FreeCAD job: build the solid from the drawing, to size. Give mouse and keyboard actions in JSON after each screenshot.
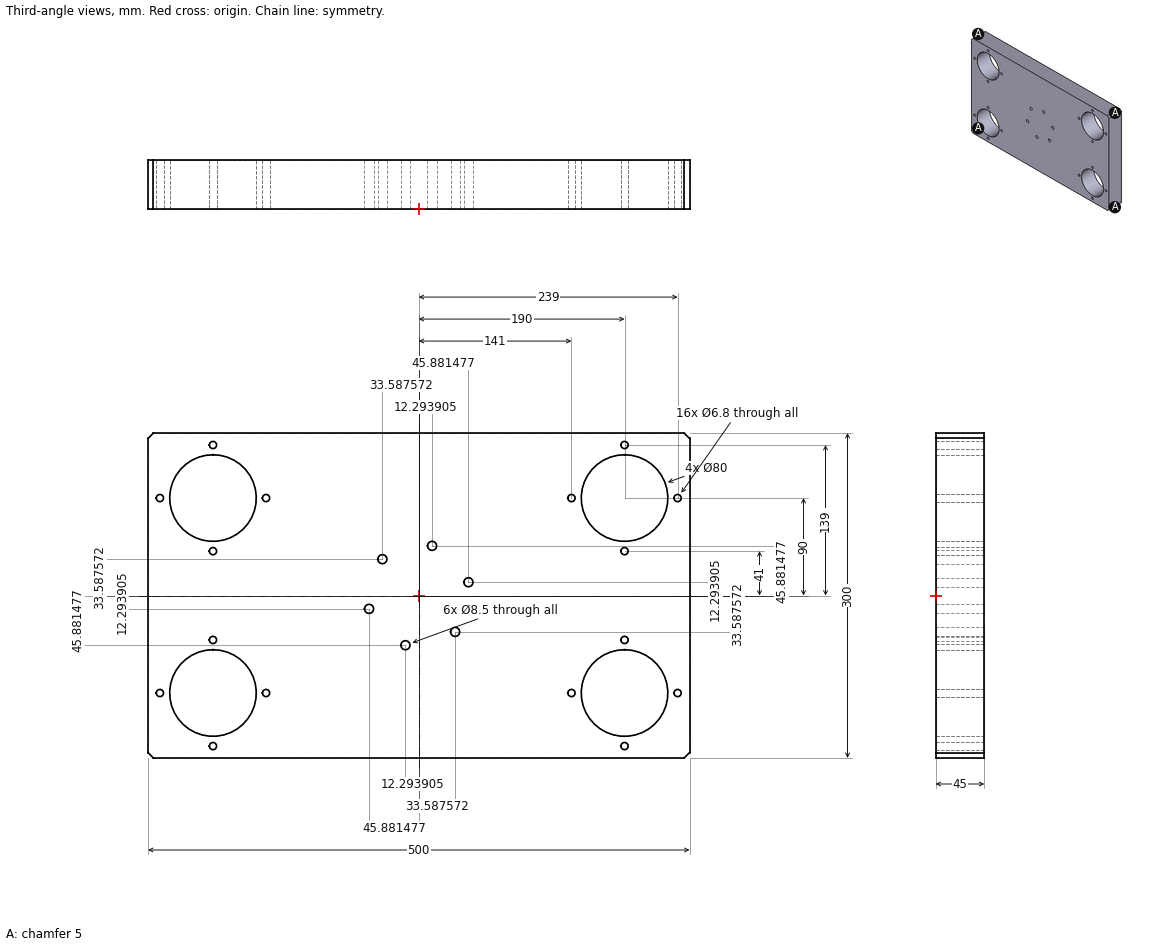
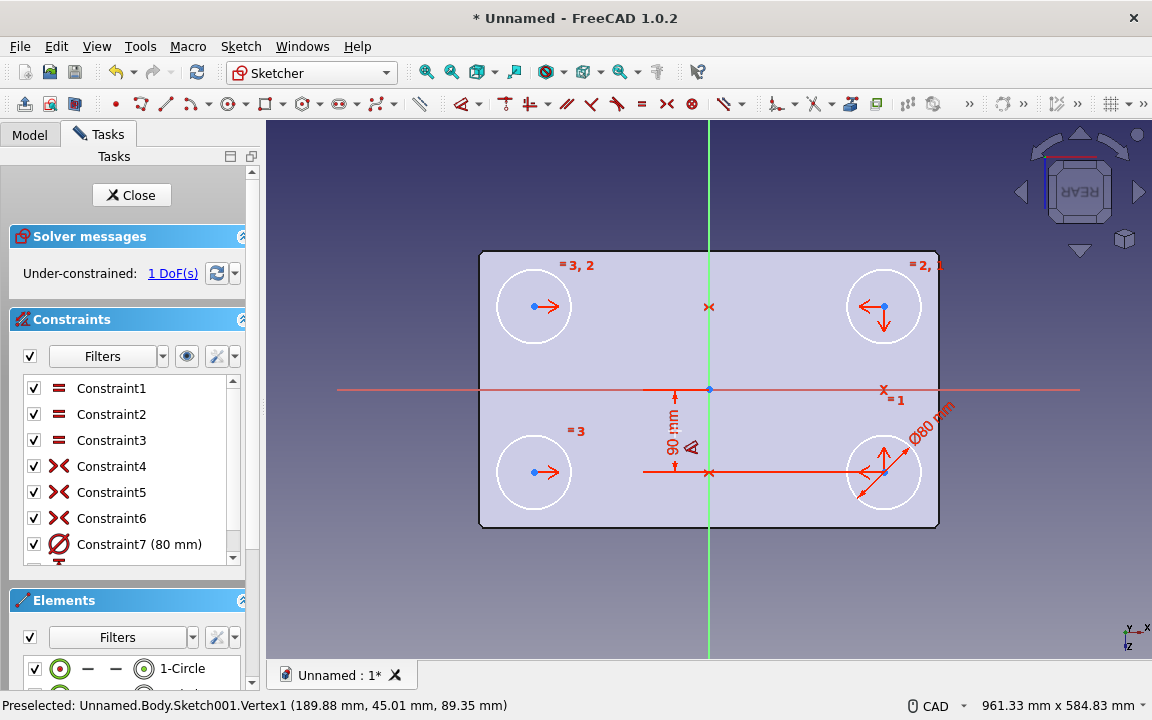
{"action": "left_click", "coordinate": [884, 472]}
{"action": "left_click", "coordinate": [796, 506]}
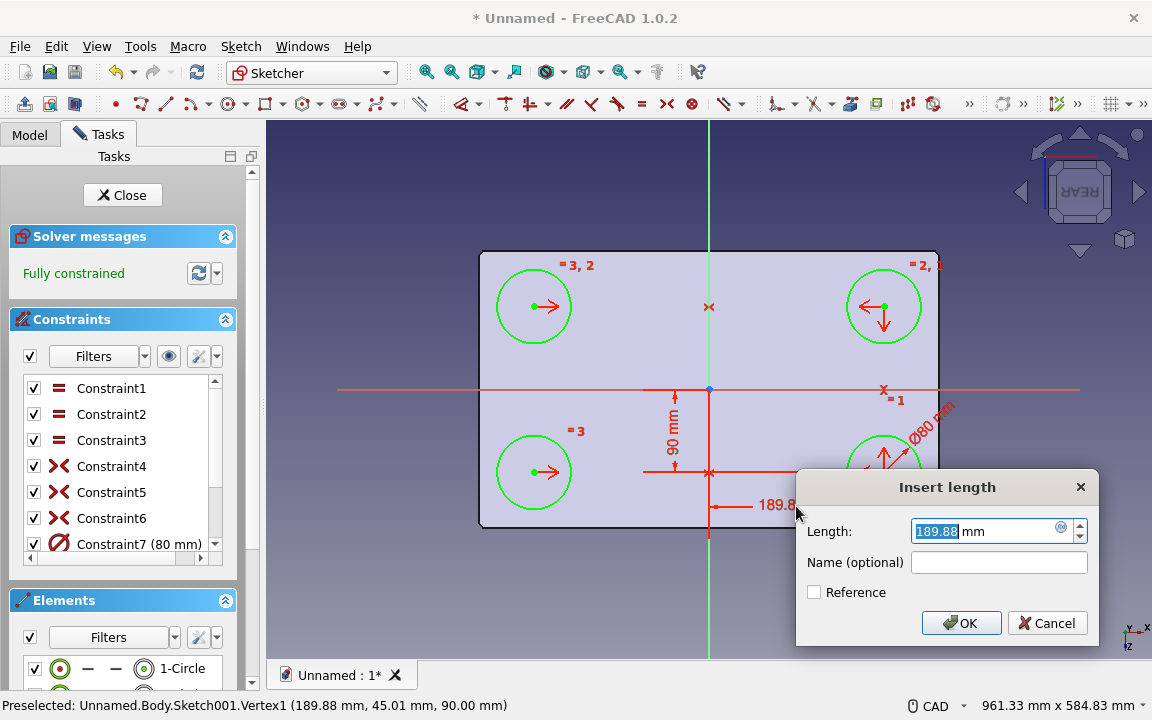
{"action": "type", "text": "190"}
{"action": "key", "text": "Return"}
{"action": "key", "text": "Escape"}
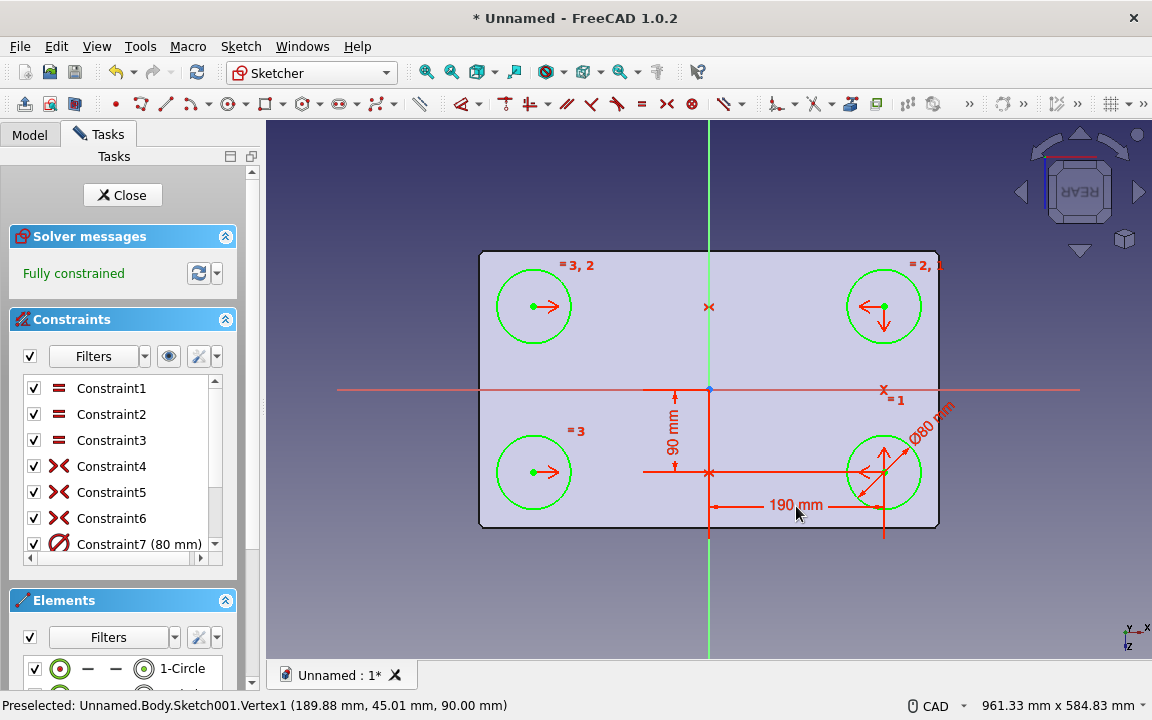
{"action": "left_click", "coordinate": [123, 195]}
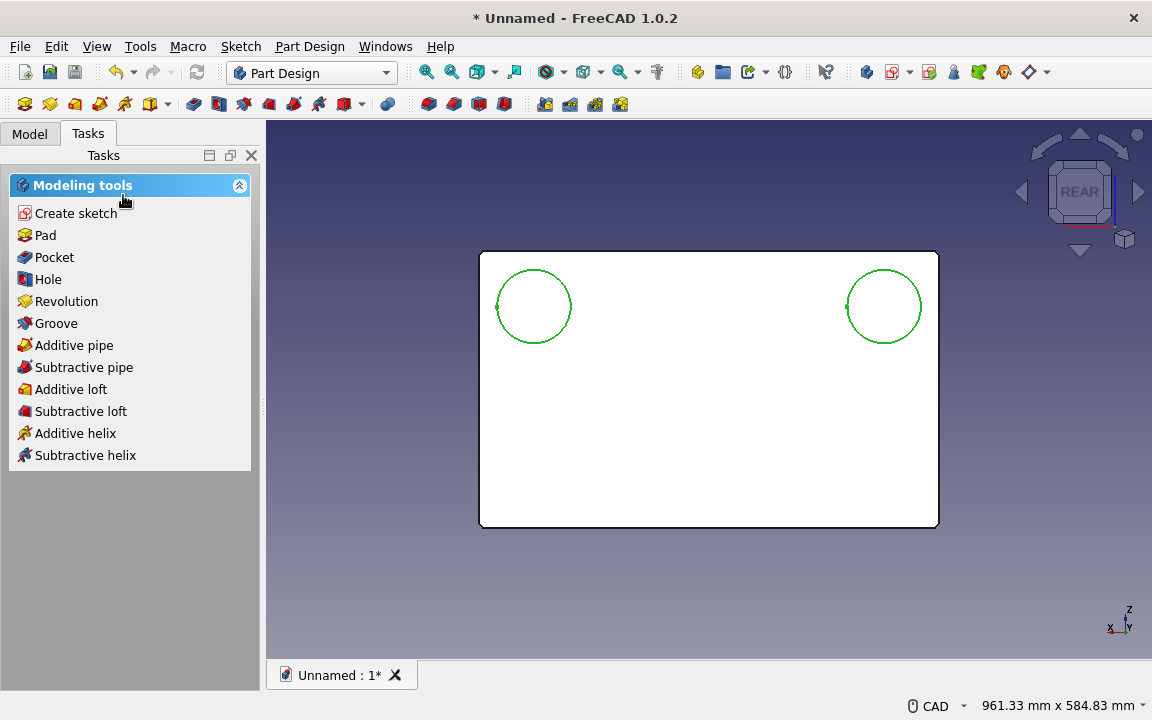
{"action": "left_click", "coordinate": [194, 104]}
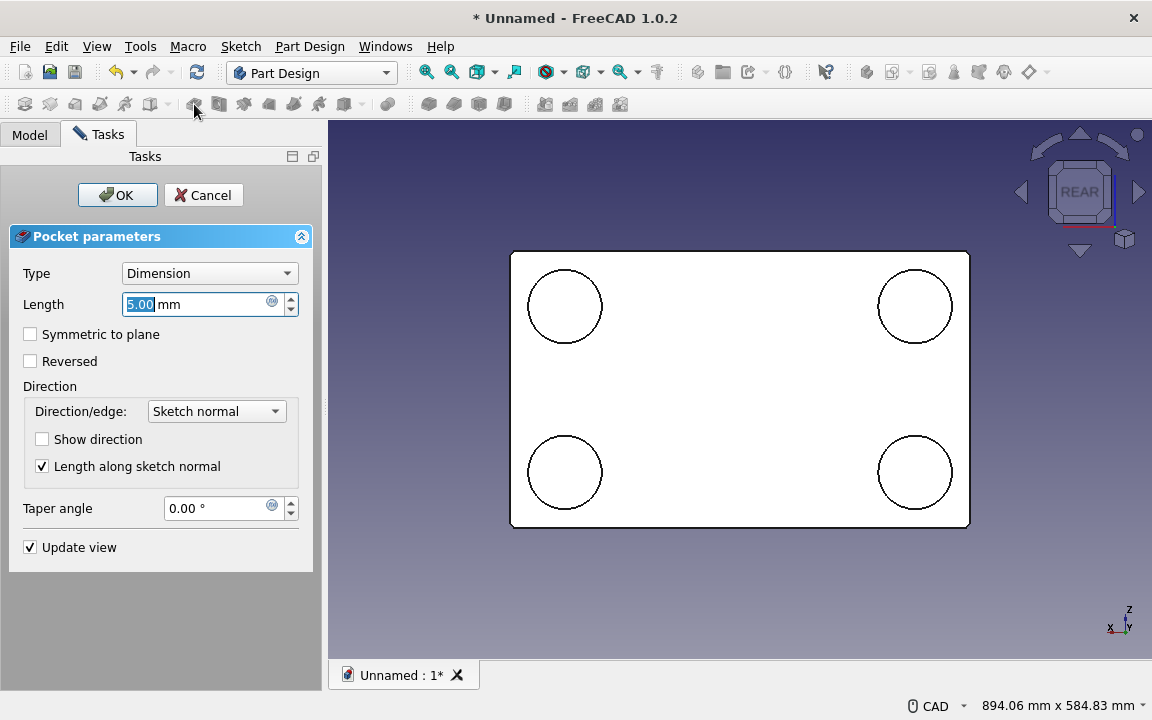
{"action": "left_click", "coordinate": [210, 274]}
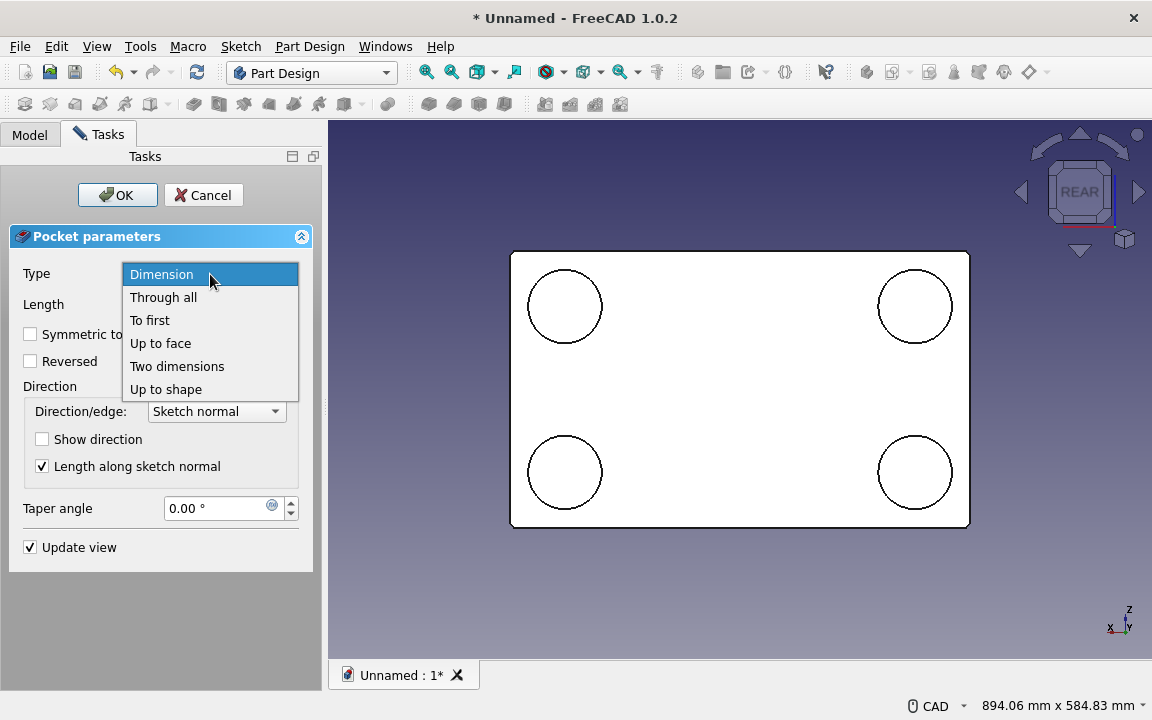
{"action": "left_click", "coordinate": [208, 298]}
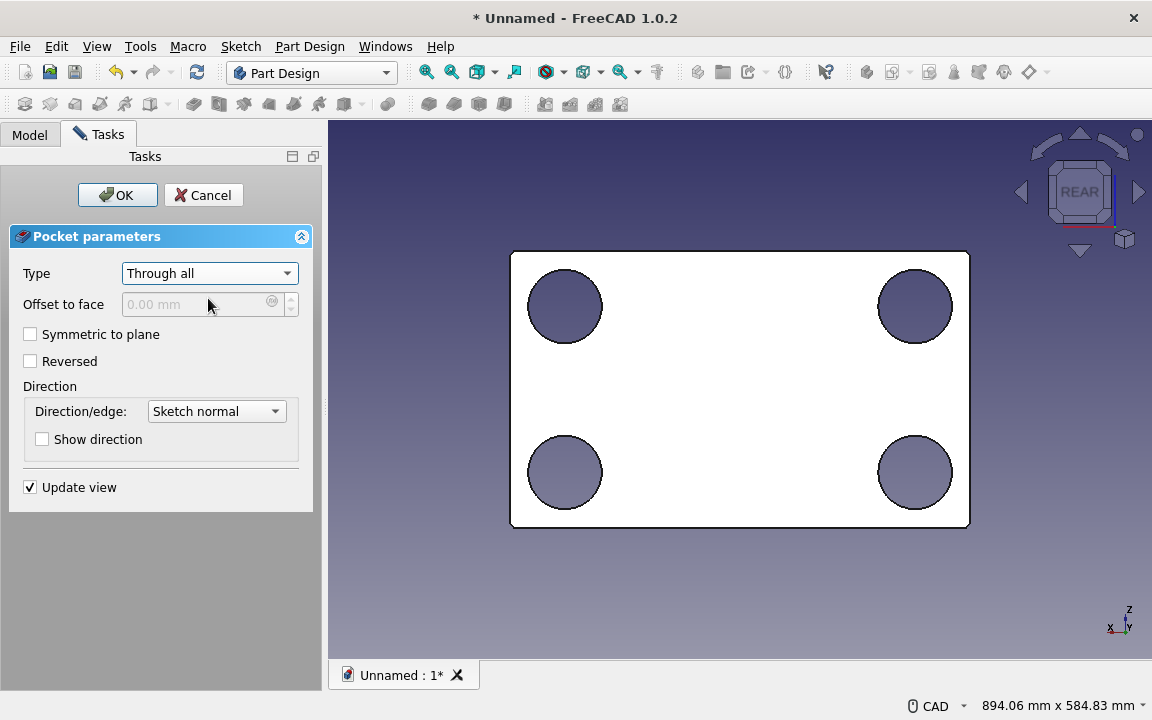
{"action": "left_click", "coordinate": [118, 195]}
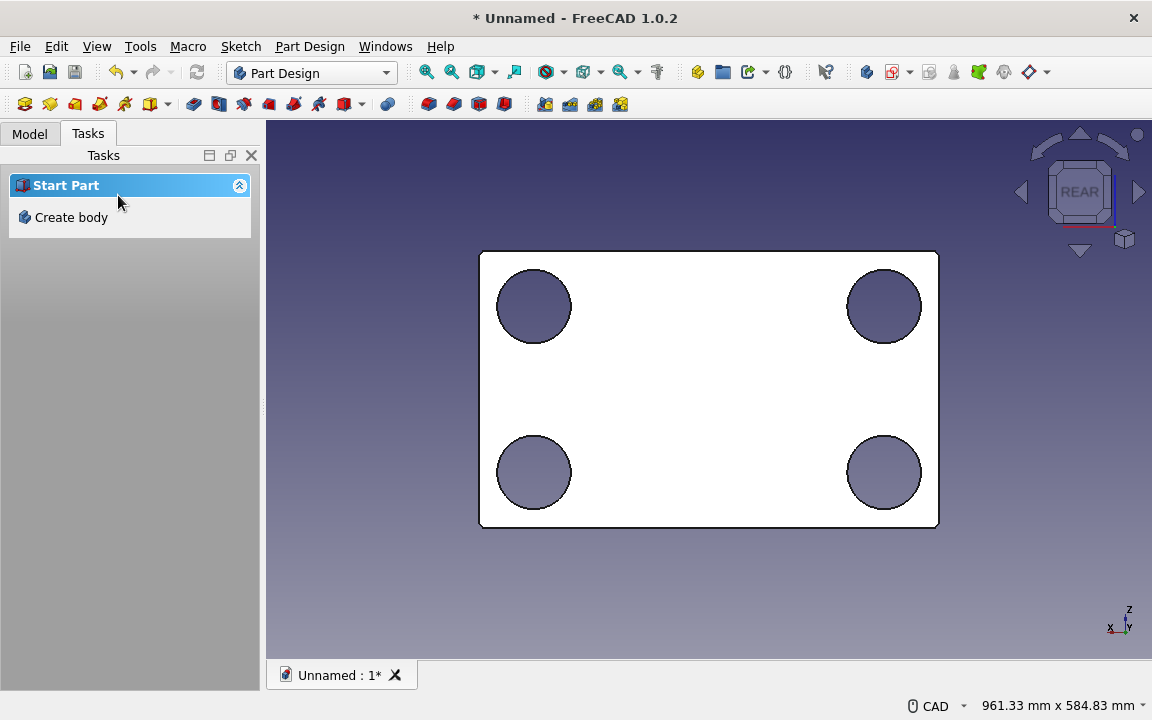
{"action": "left_click", "coordinate": [709, 389]}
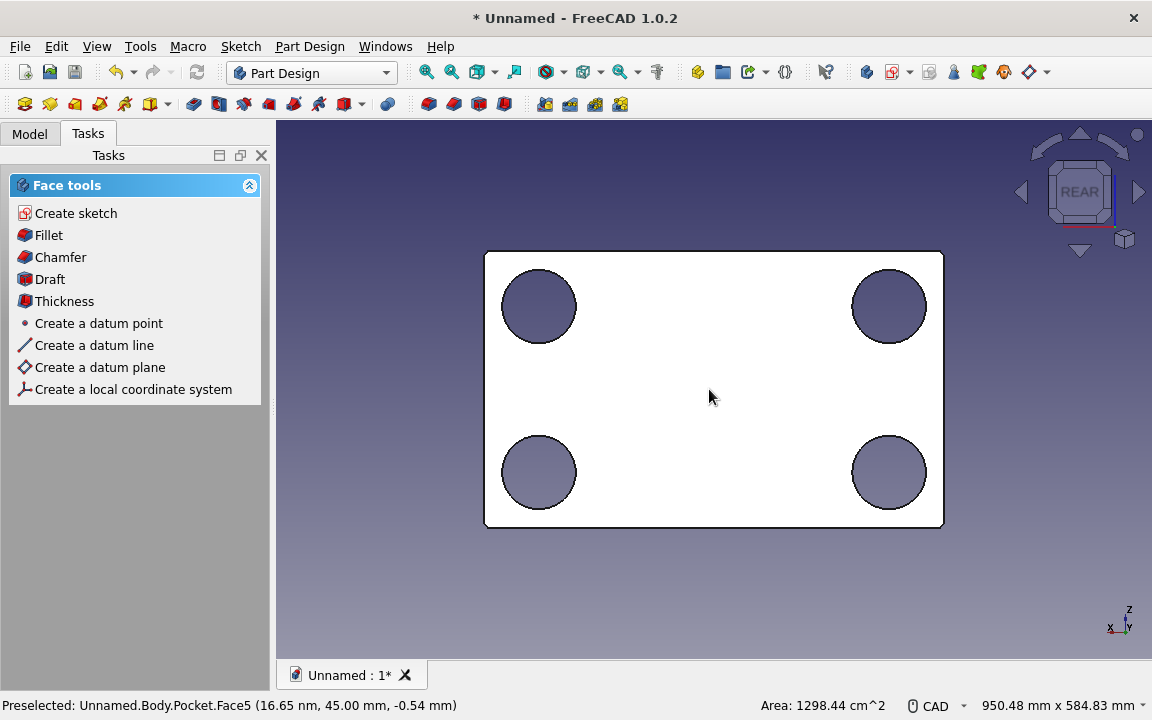
{"action": "left_click", "coordinate": [892, 72]}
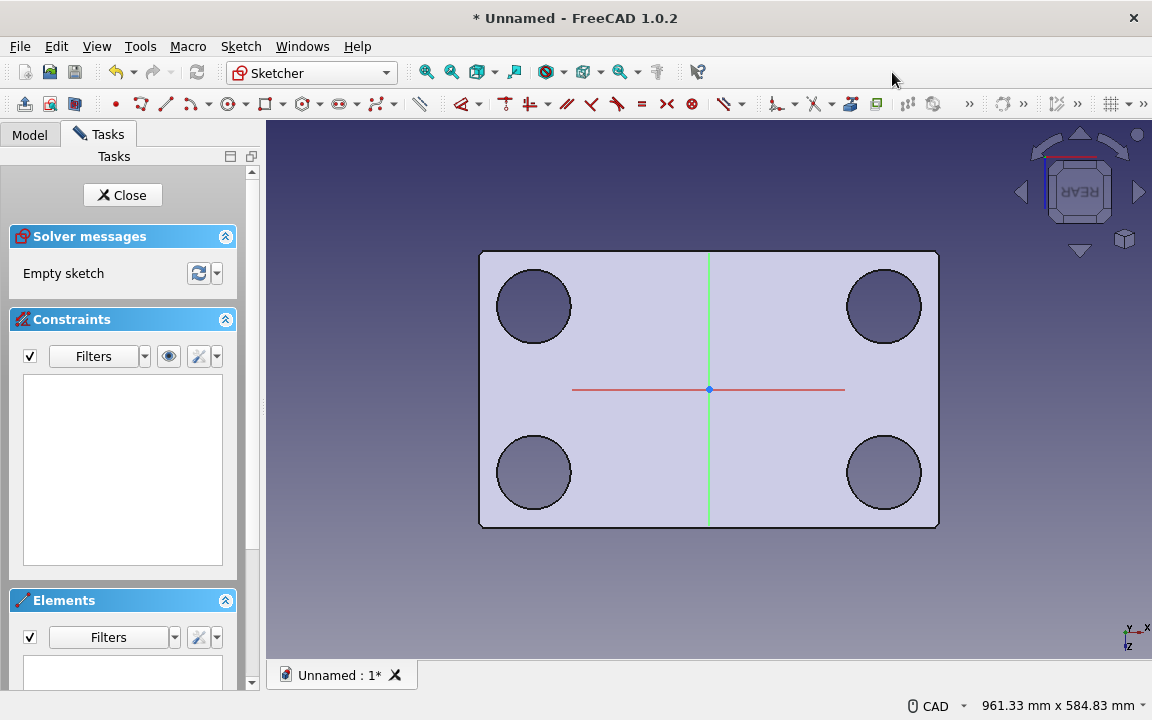
{"action": "scroll", "coordinate": [731, 389], "scroll_direction": "up", "scroll_amount": 7}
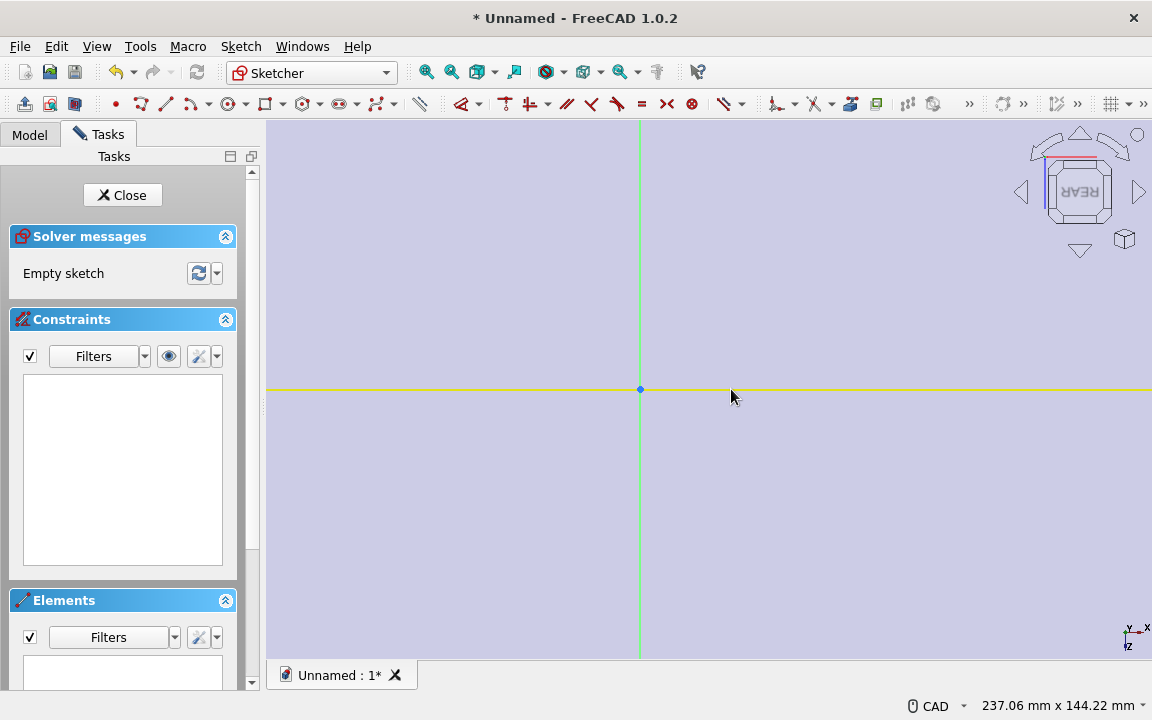
{"action": "left_click", "coordinate": [228, 104]}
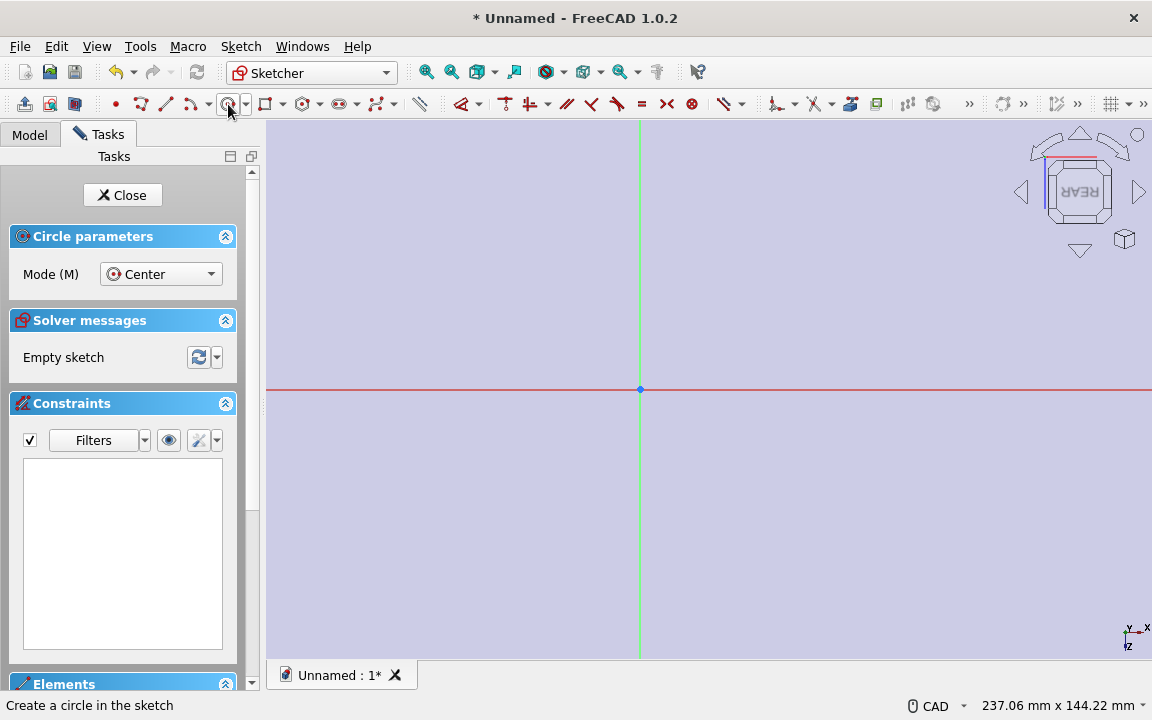
{"action": "scroll", "coordinate": [594, 218], "scroll_direction": "up", "scroll_amount": 2}